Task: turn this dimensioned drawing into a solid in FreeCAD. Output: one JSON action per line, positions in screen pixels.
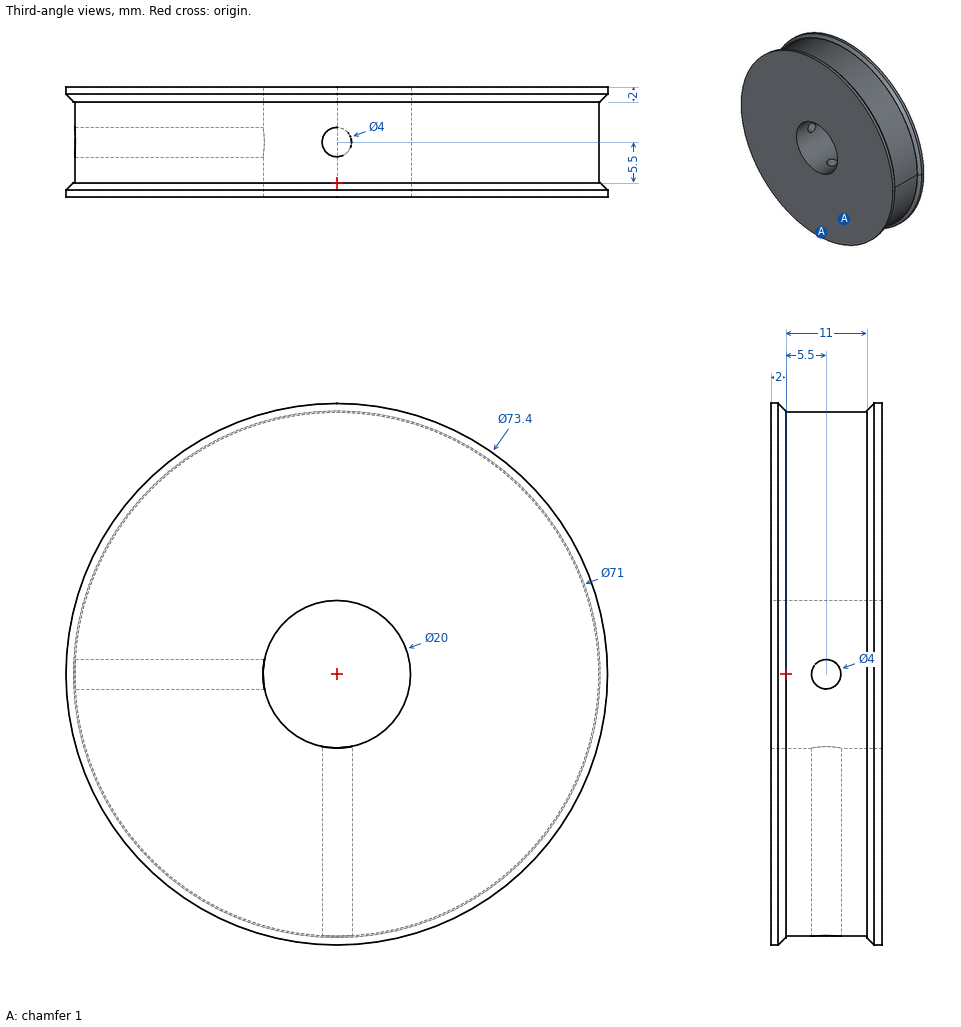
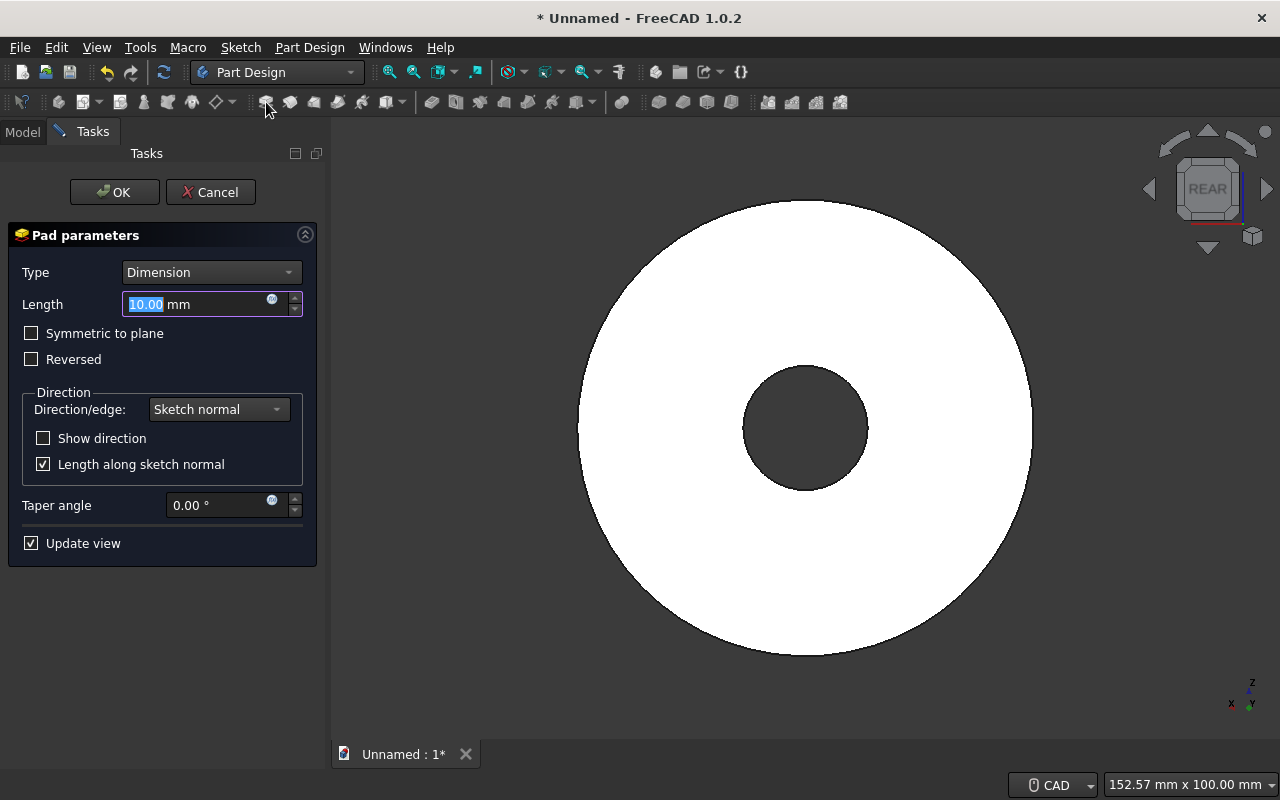
{"action": "type", "text": "2"}
{"action": "key", "text": "Tab"}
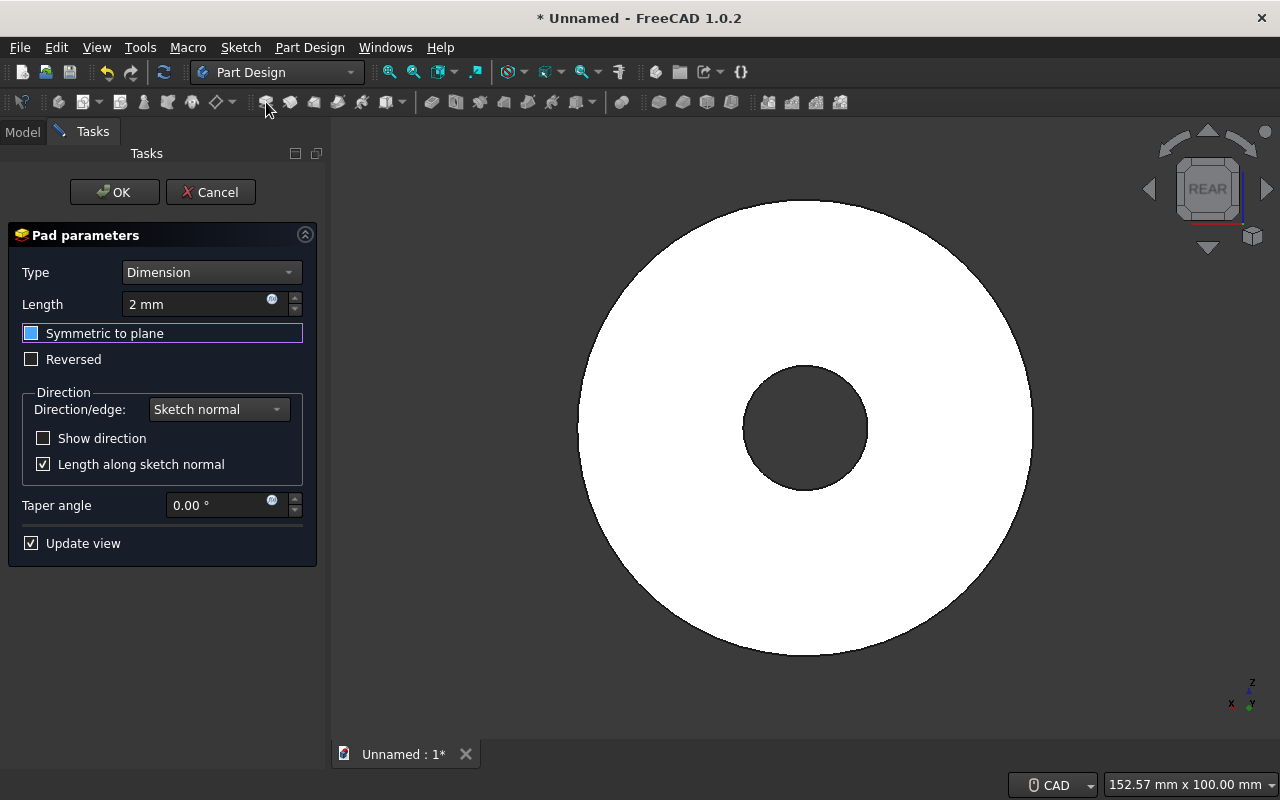
{"action": "left_click", "coordinate": [115, 192]}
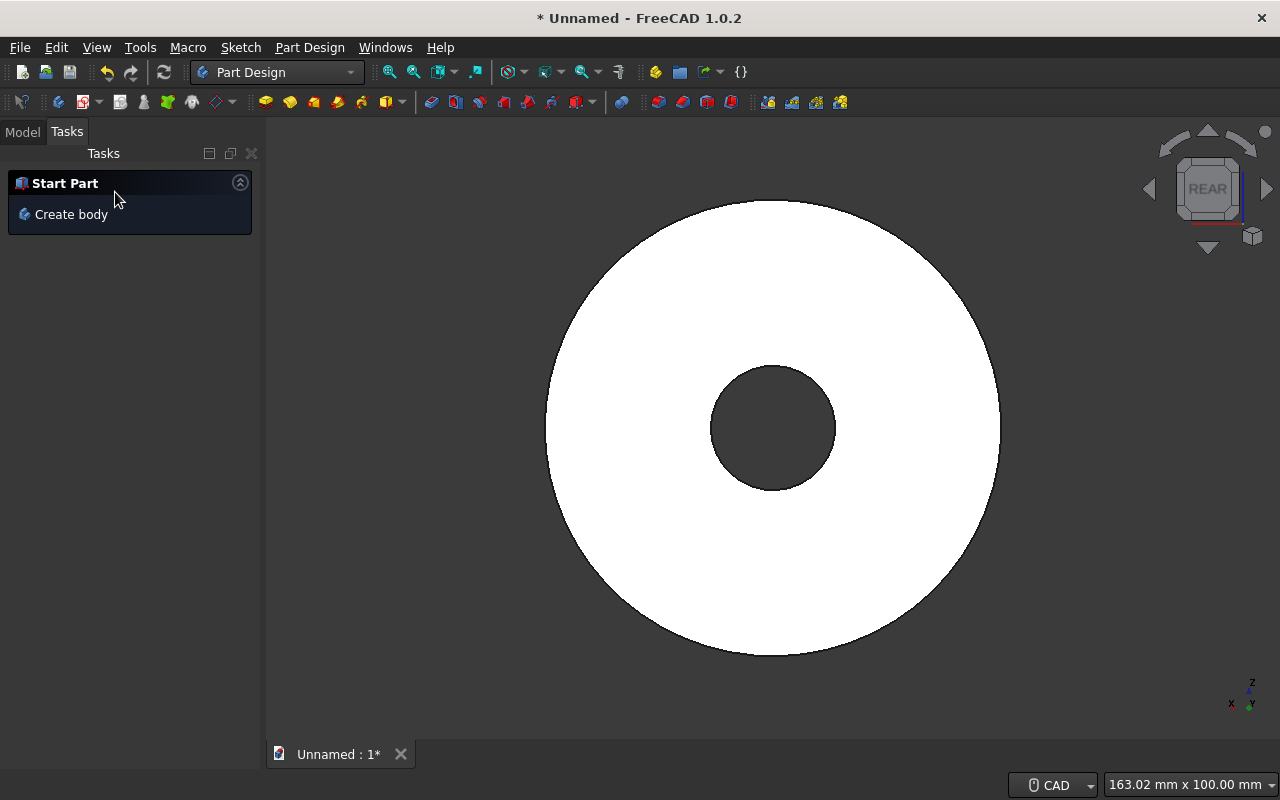
{"action": "left_click", "coordinate": [23, 131]}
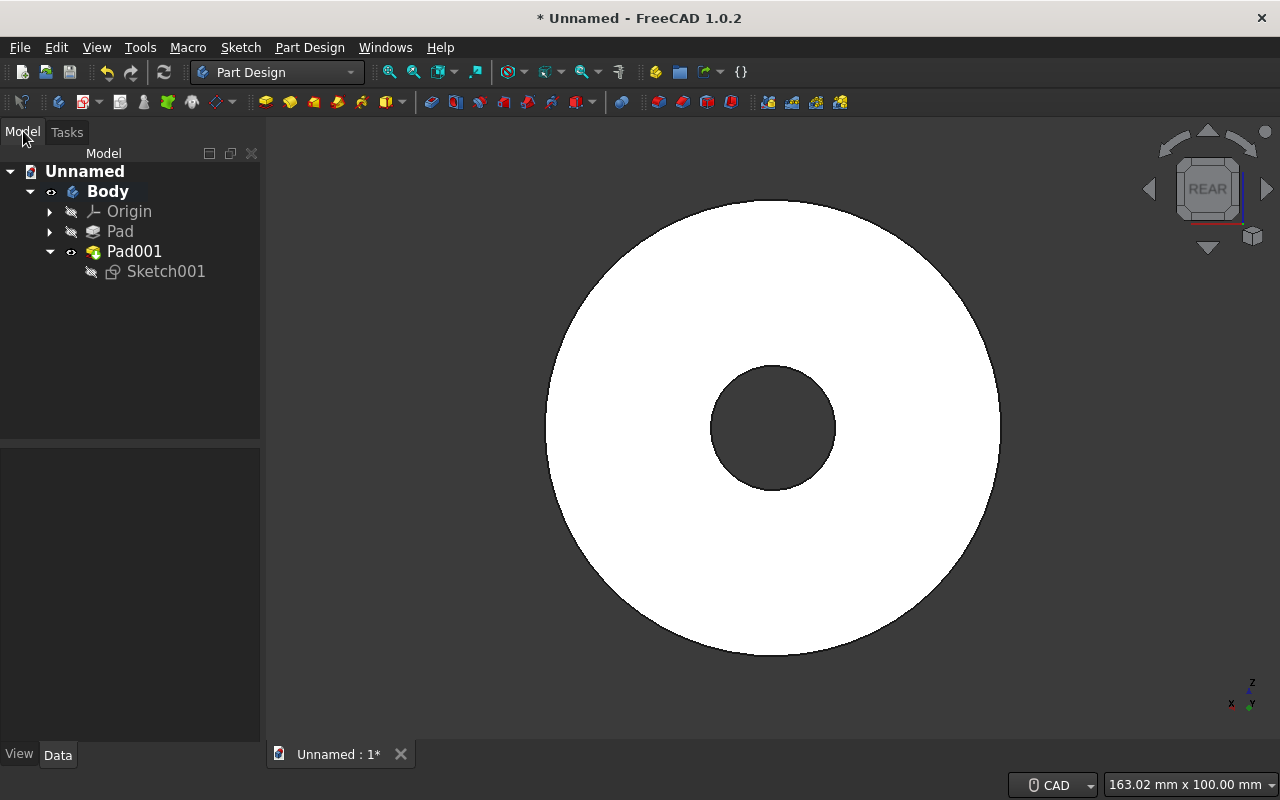
{"action": "left_click", "coordinate": [50, 212]}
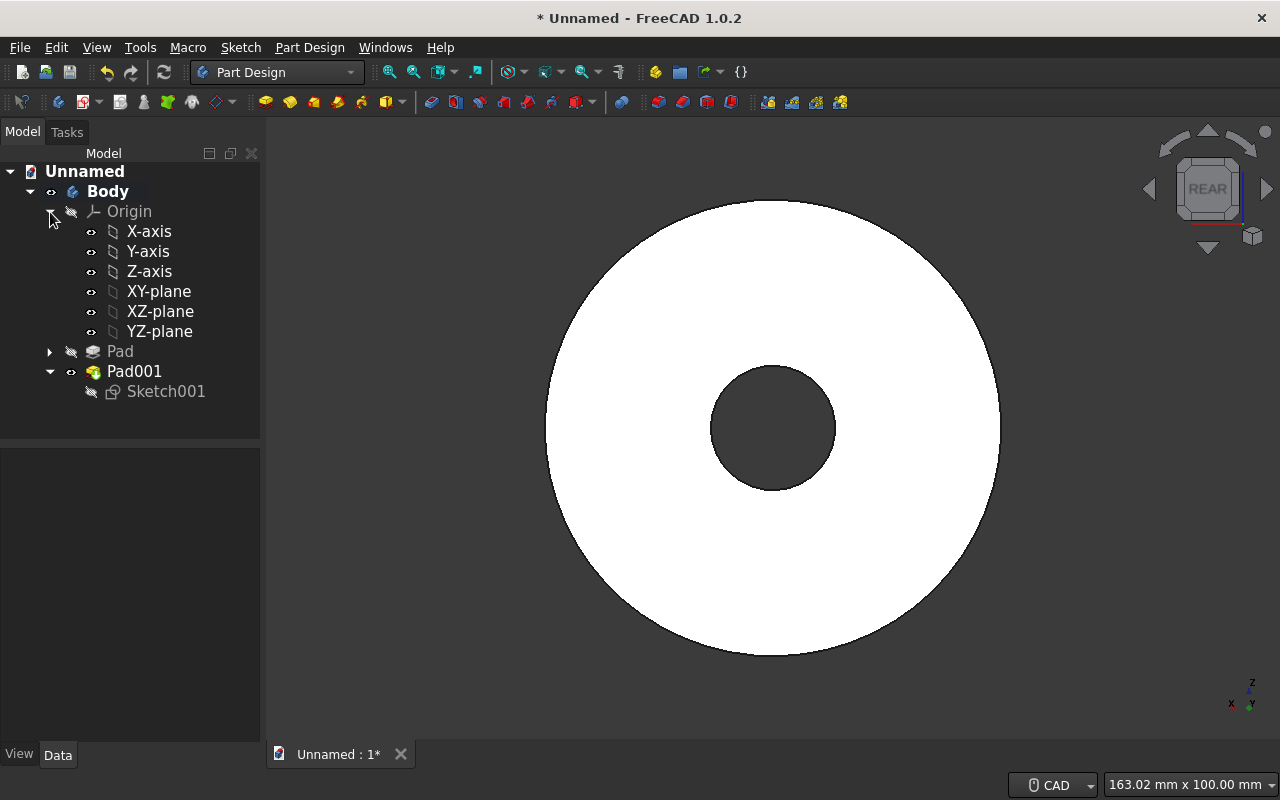
{"action": "left_click", "coordinate": [136, 312]}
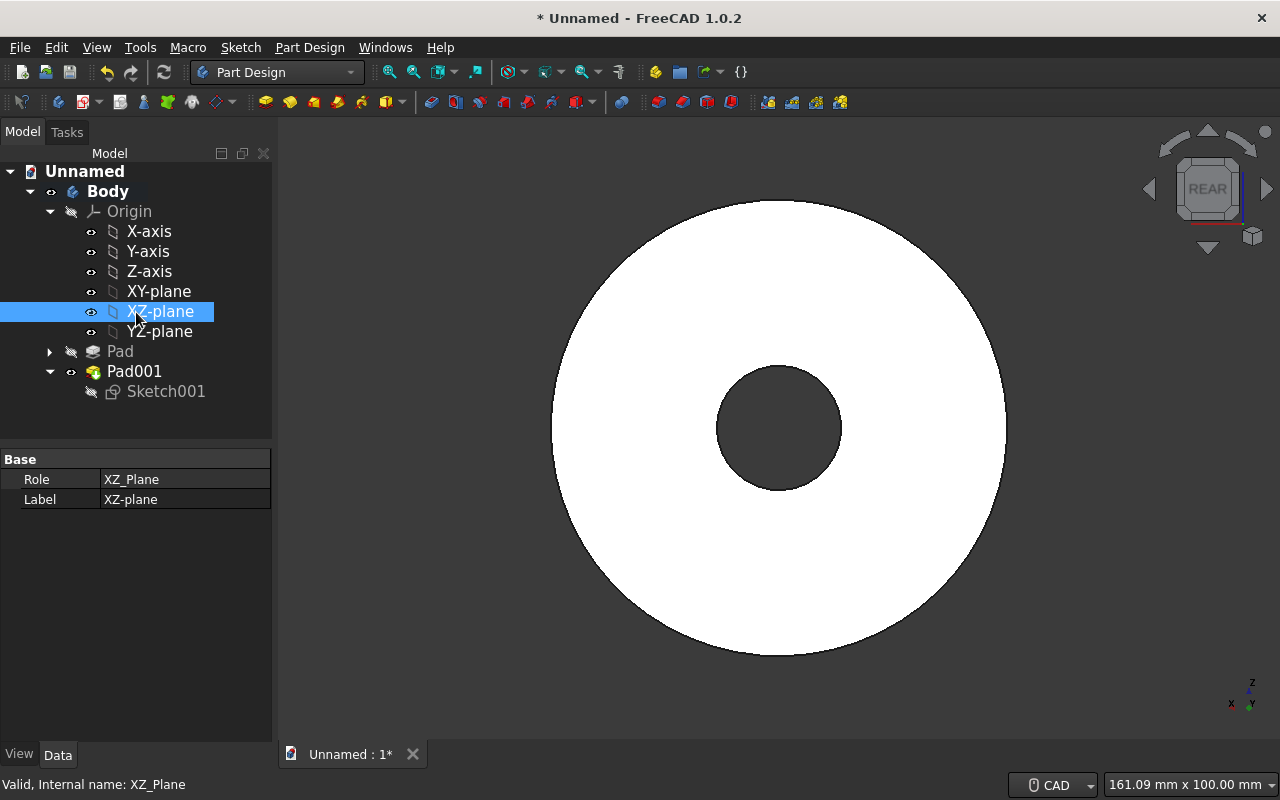
{"action": "left_click", "coordinate": [216, 102]}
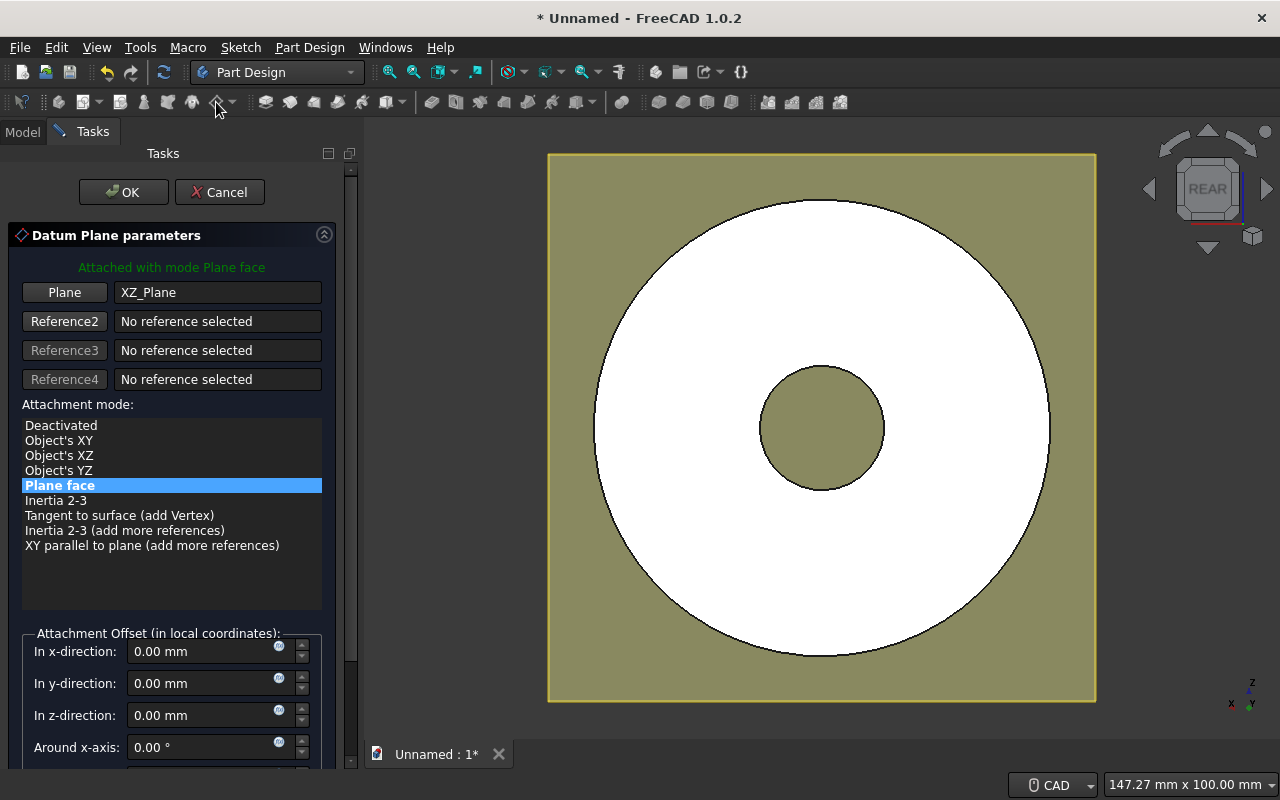
{"action": "triple_click", "coordinate": [210, 715]}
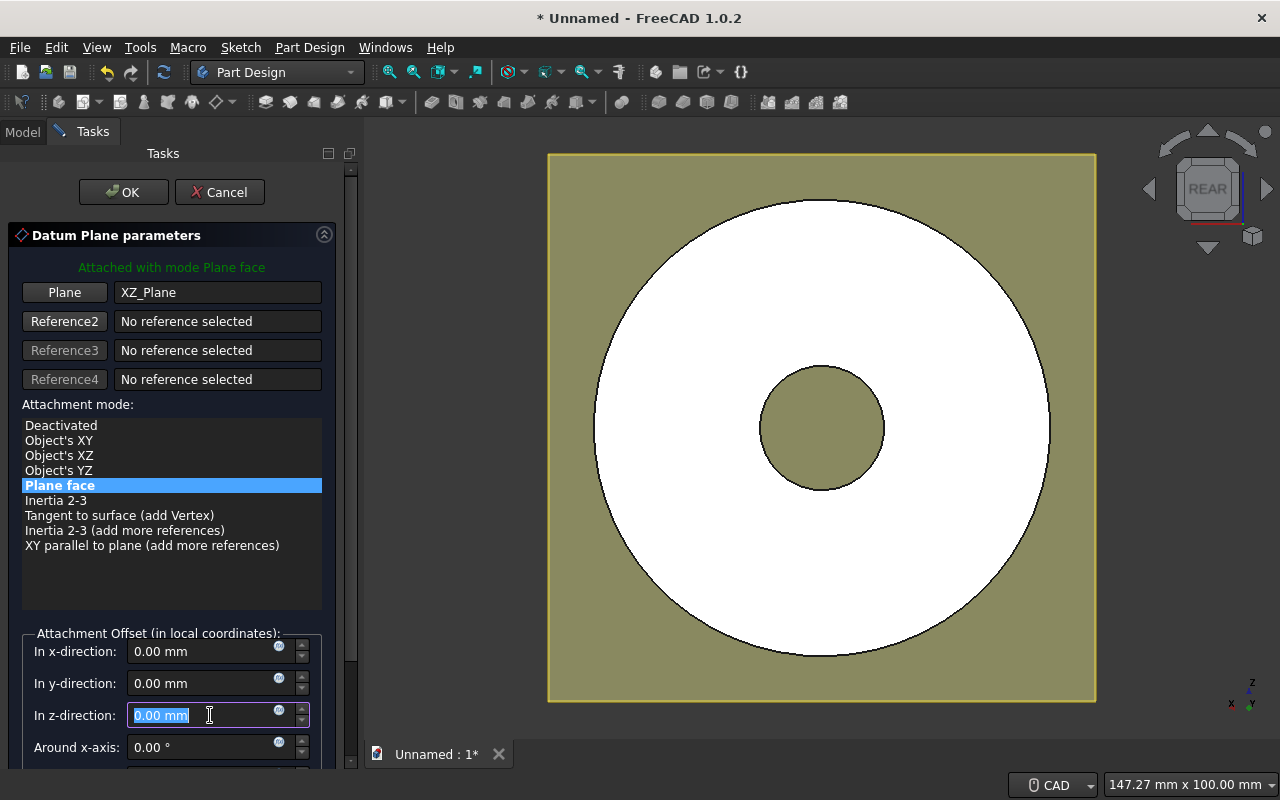
{"action": "type", "text": "2"}
{"action": "key", "text": "Tab"}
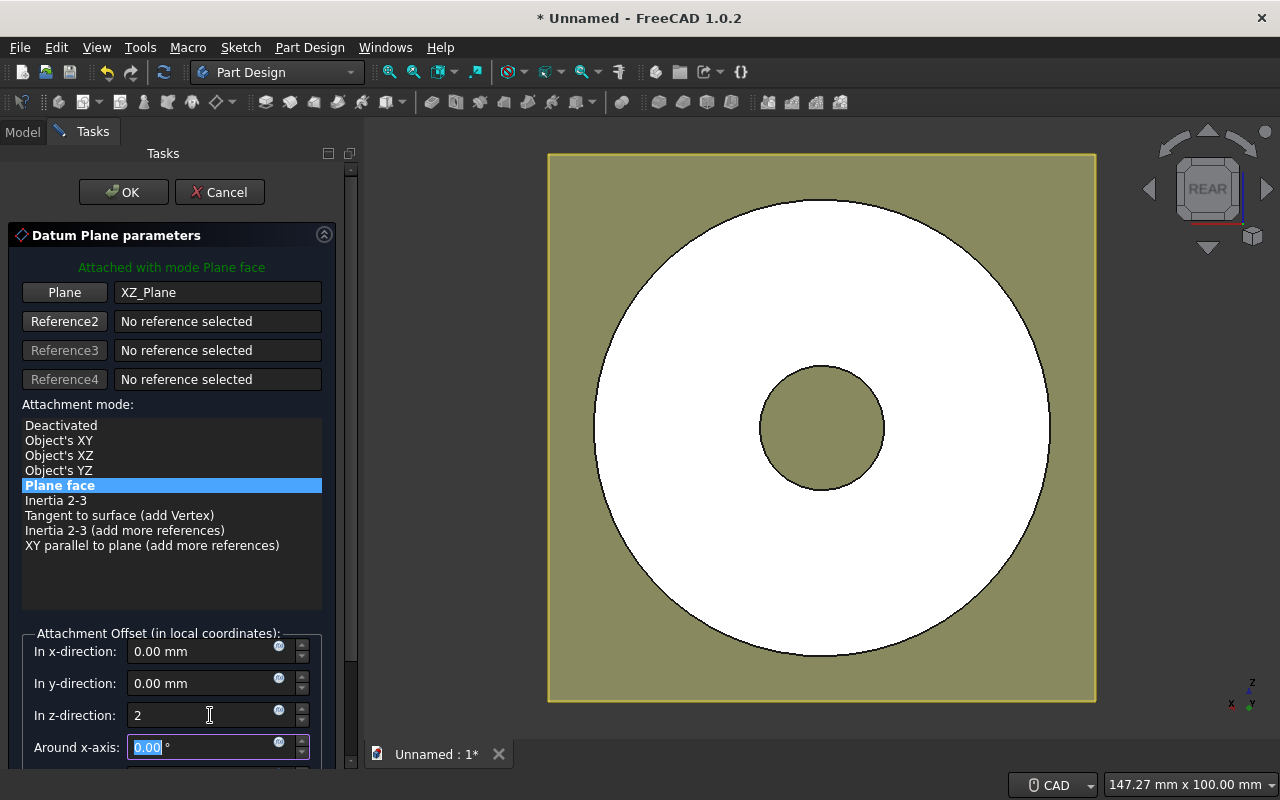
{"action": "left_click", "coordinate": [124, 192]}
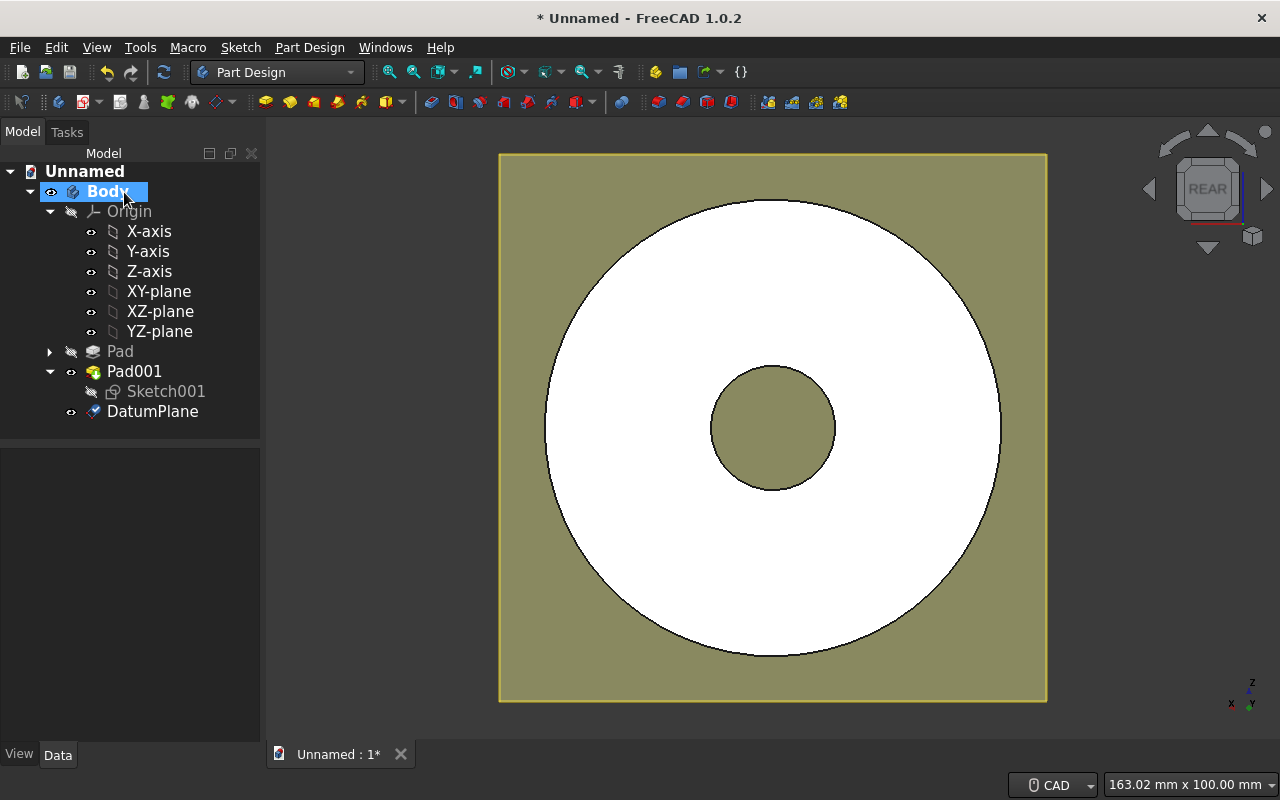
{"action": "left_click", "coordinate": [116, 412]}